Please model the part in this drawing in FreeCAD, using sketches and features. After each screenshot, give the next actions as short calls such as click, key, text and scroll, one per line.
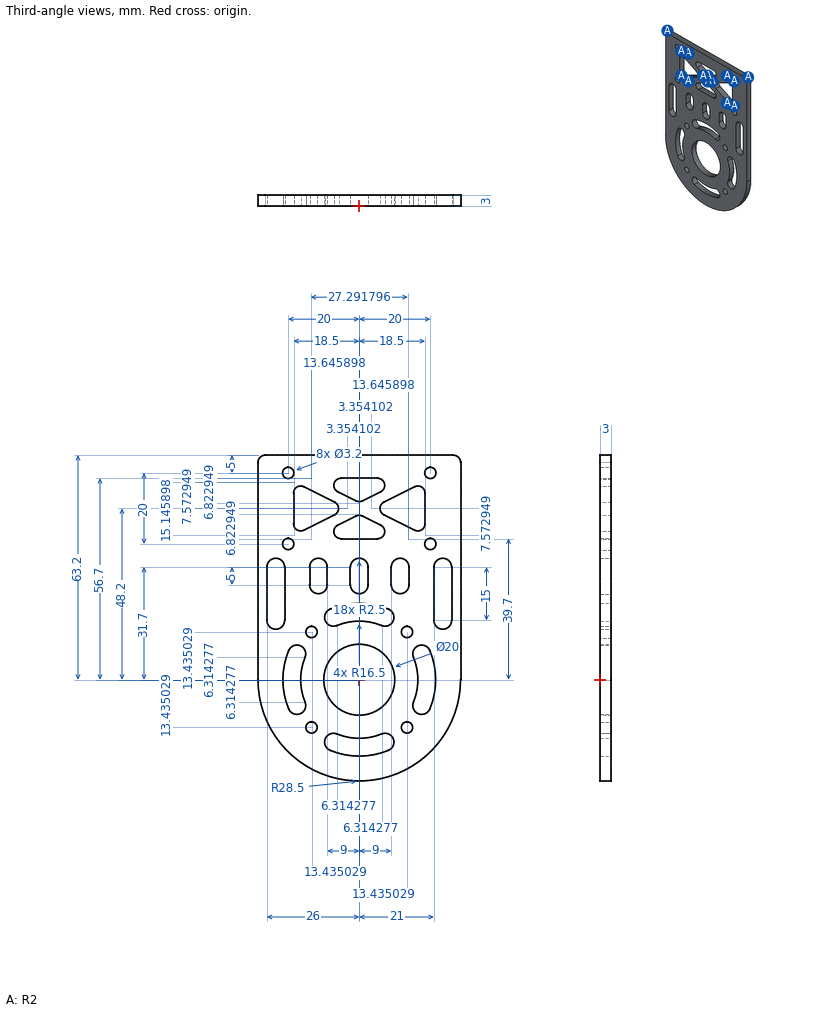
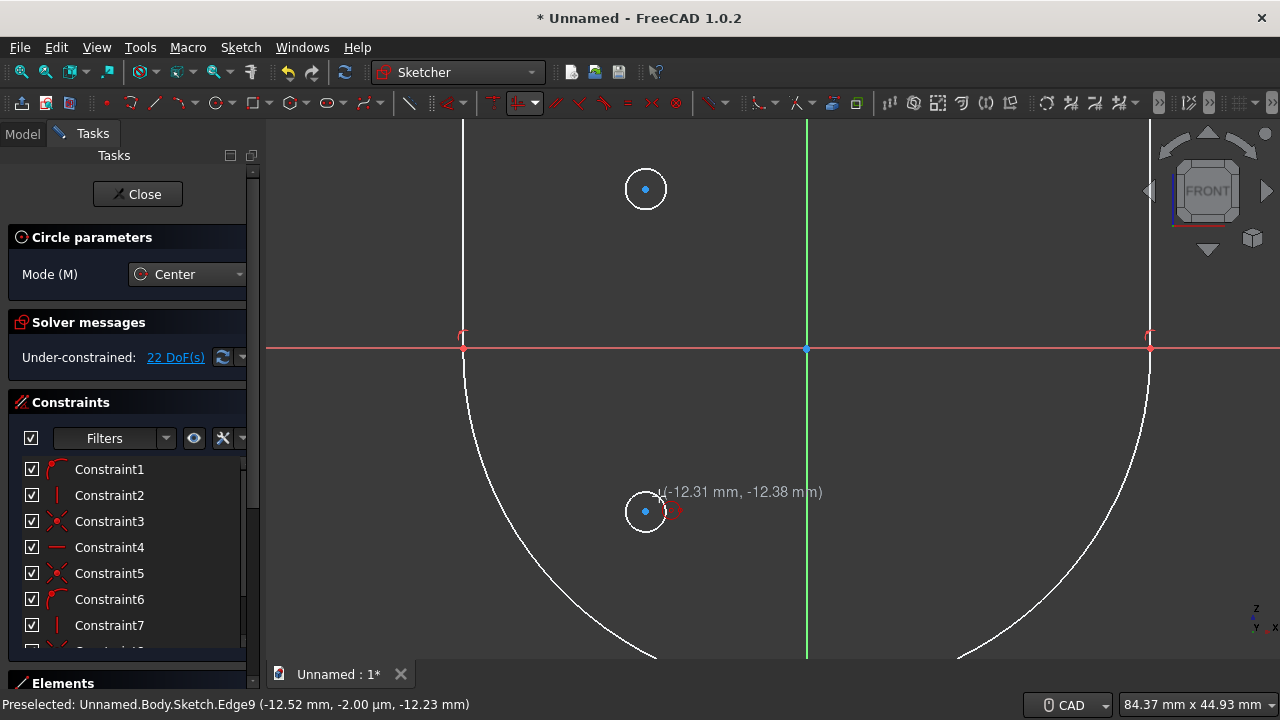
click(968, 187)
click(982, 173)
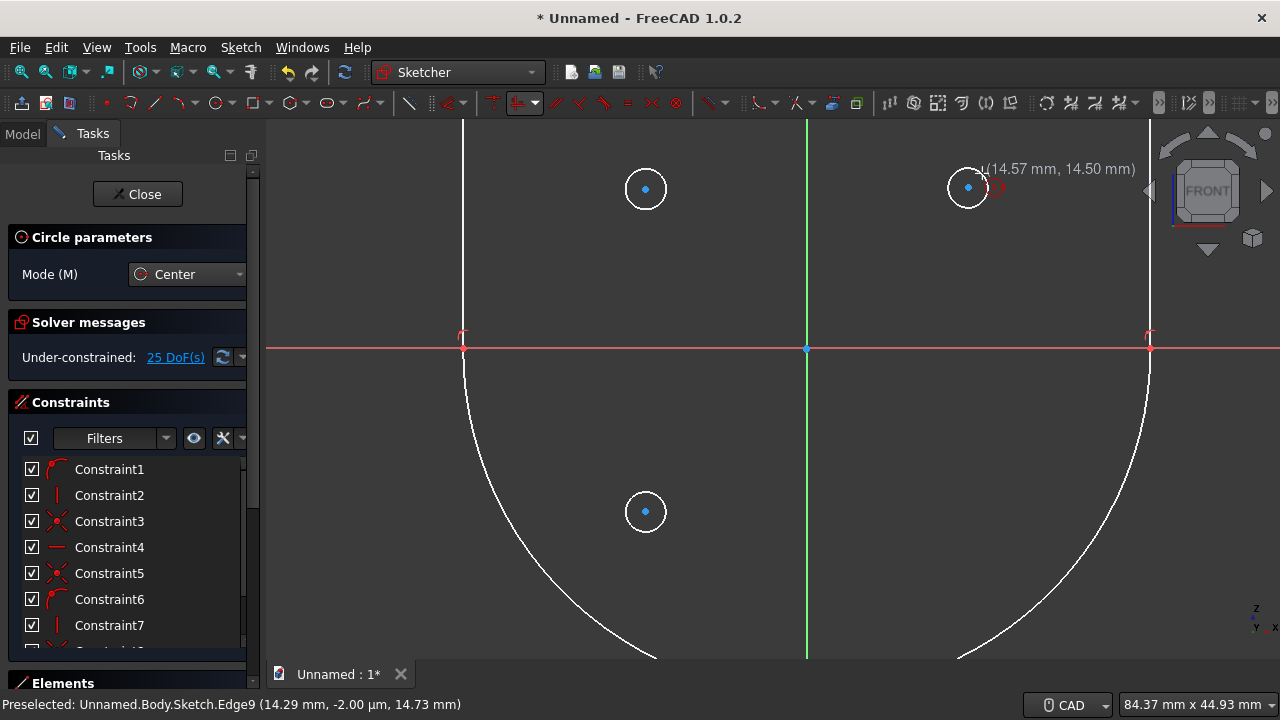
click(807, 348)
click(892, 263)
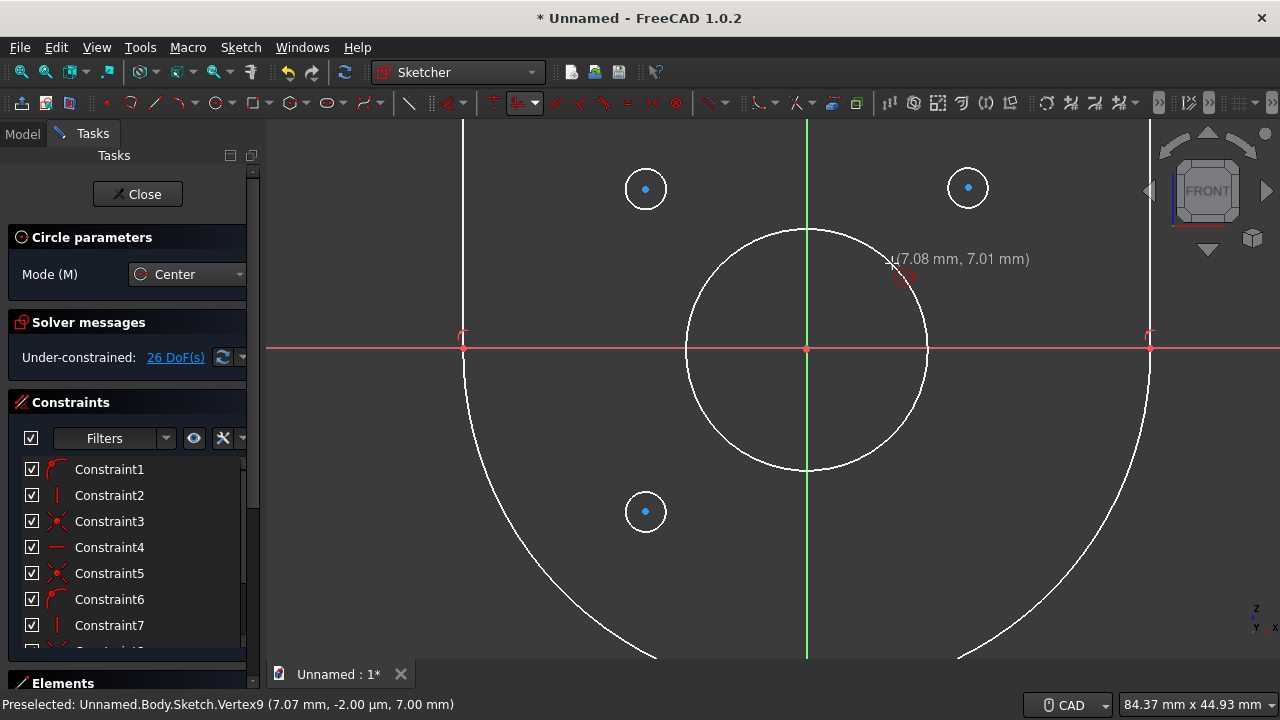
click(968, 510)
click(982, 496)
key(Escape)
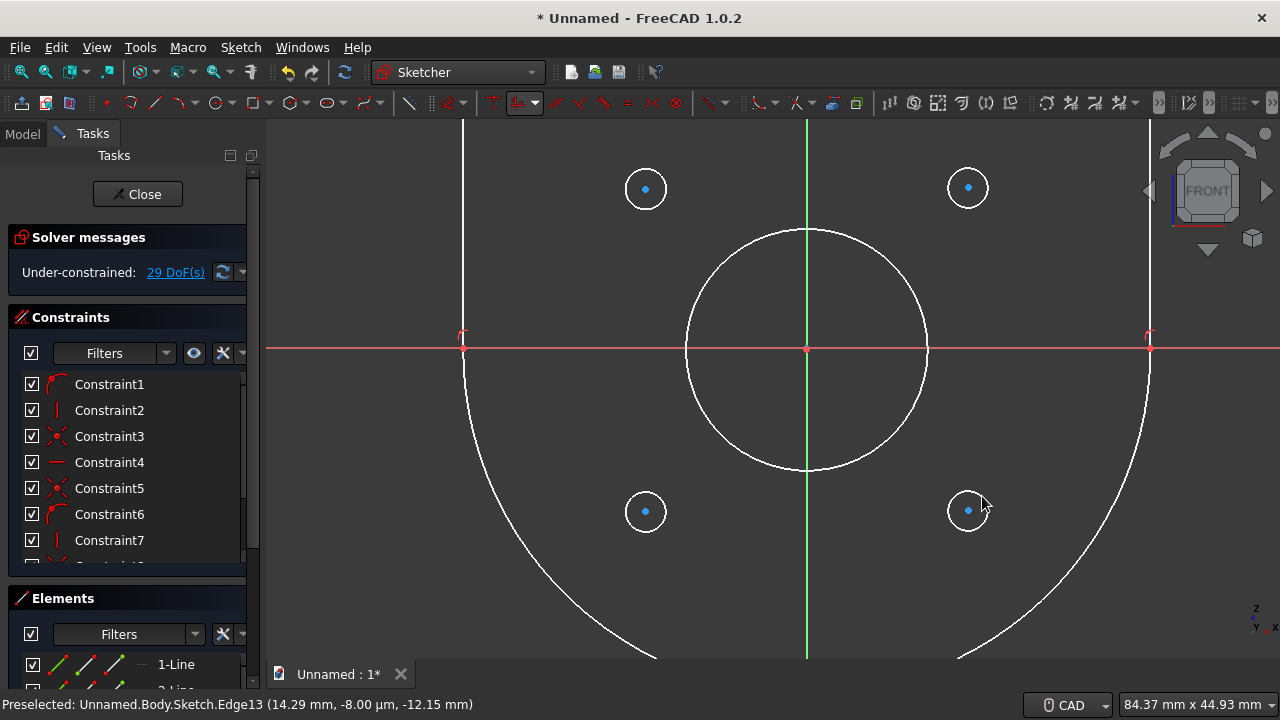
scroll(807, 349, up, 4)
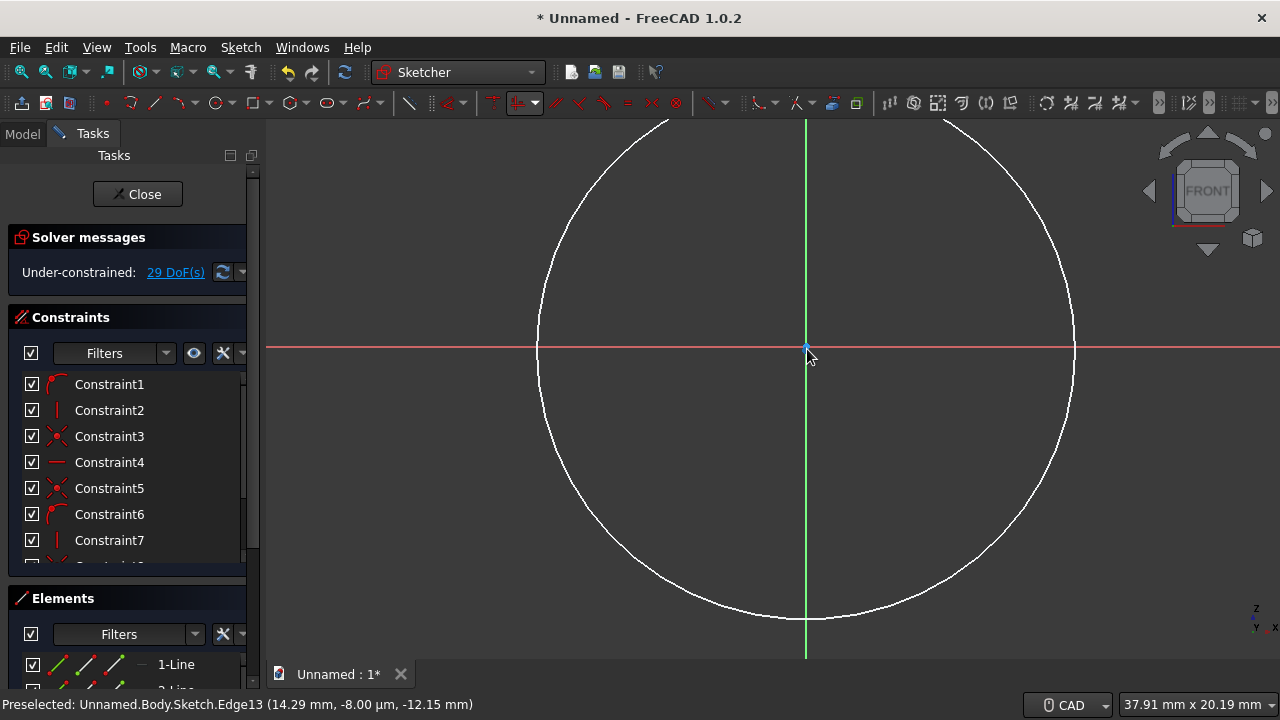
drag(796, 337, 816, 360)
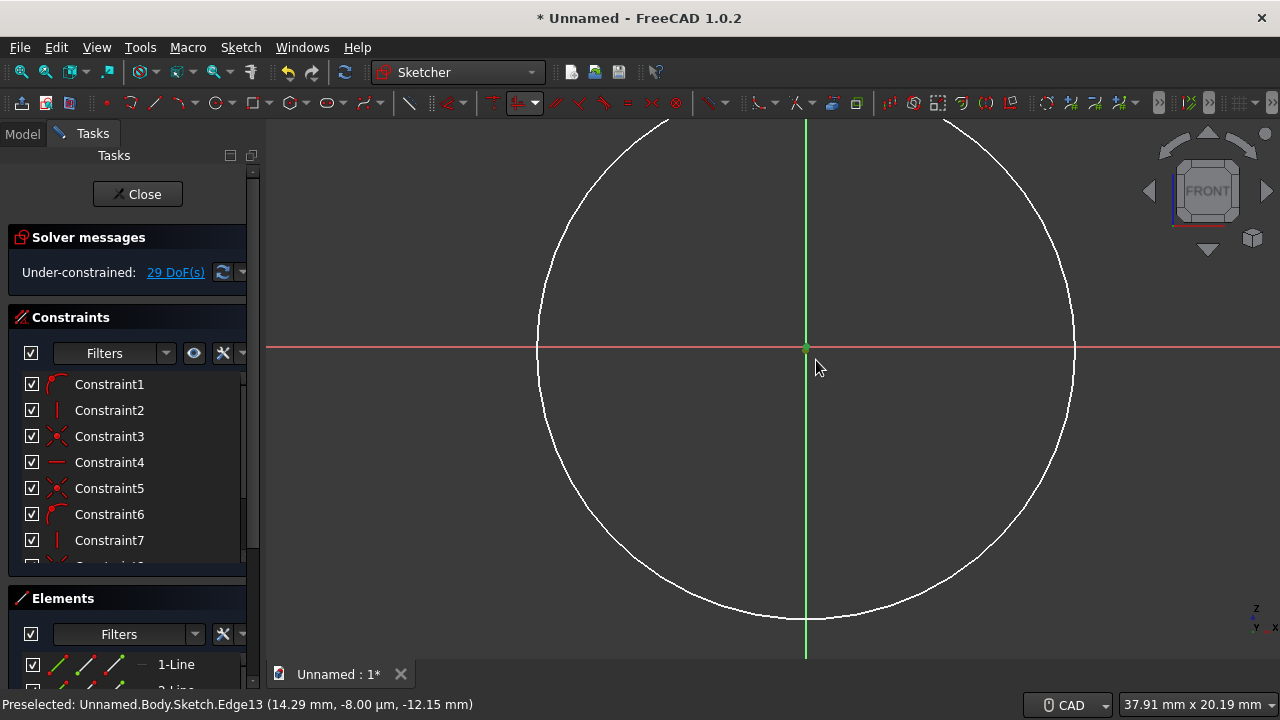
key(c)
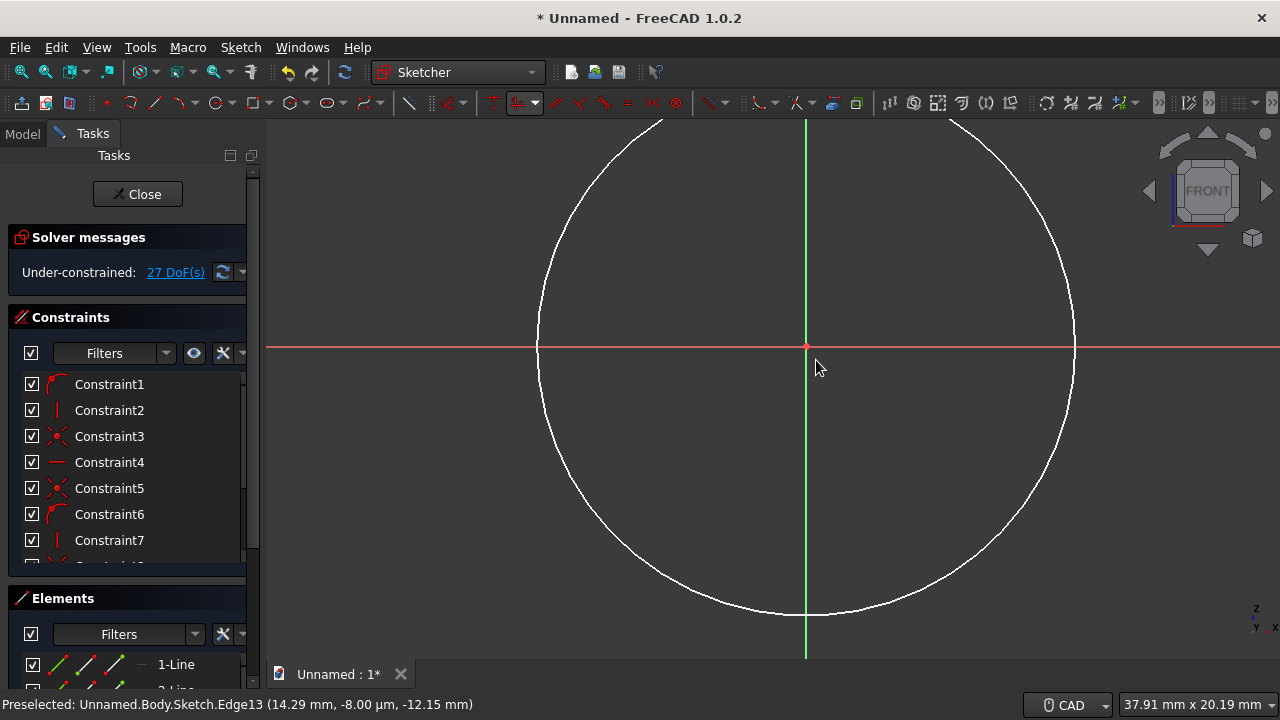
scroll(689, 468, down, 10)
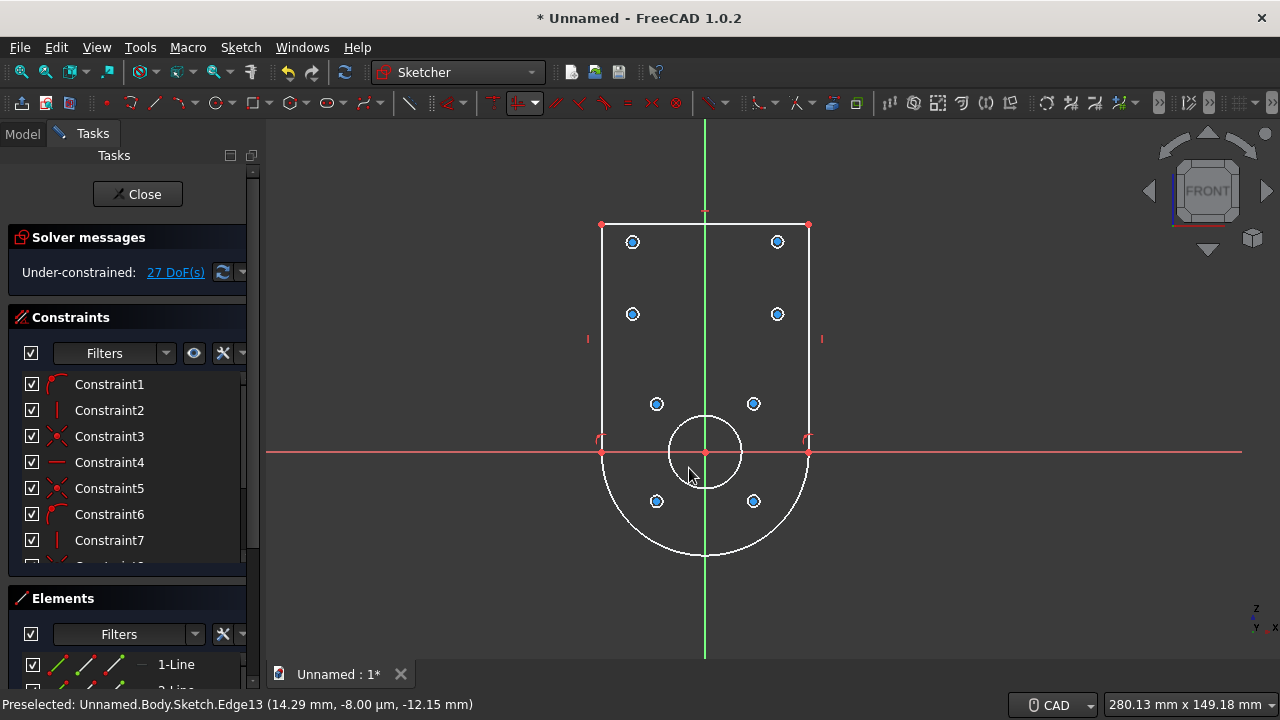
scroll(637, 238, up, 4)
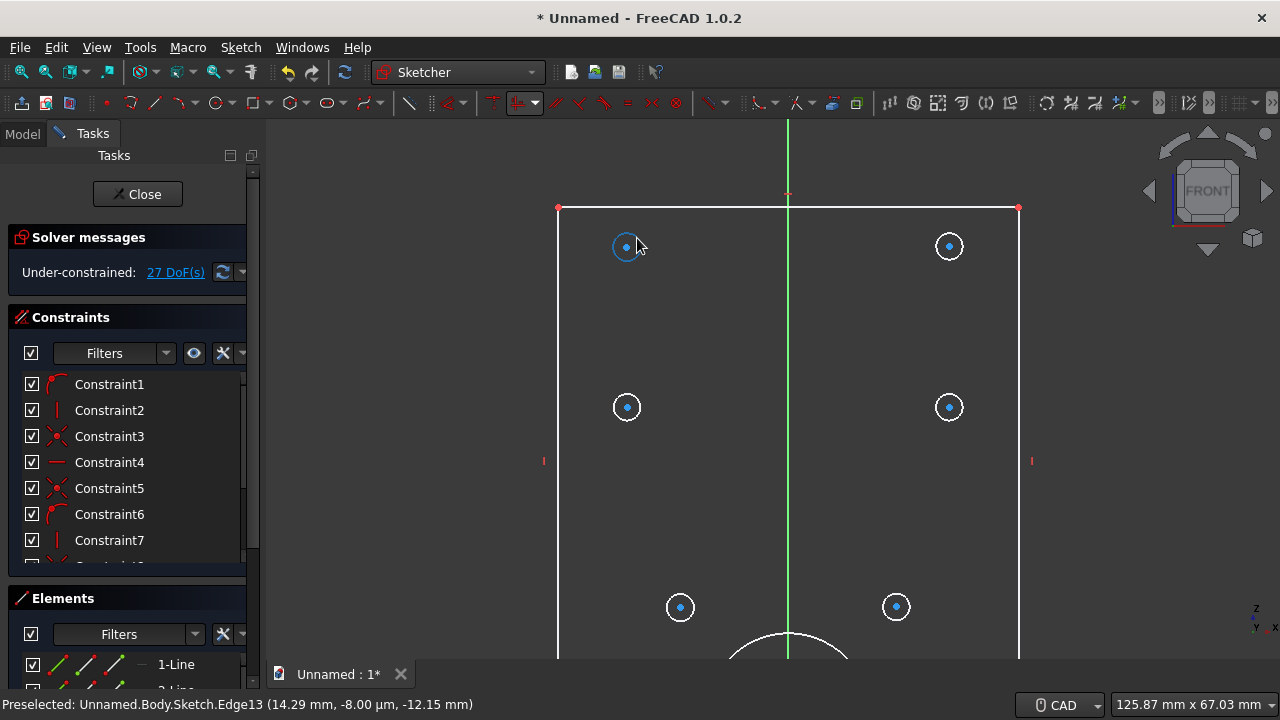
click(637, 237)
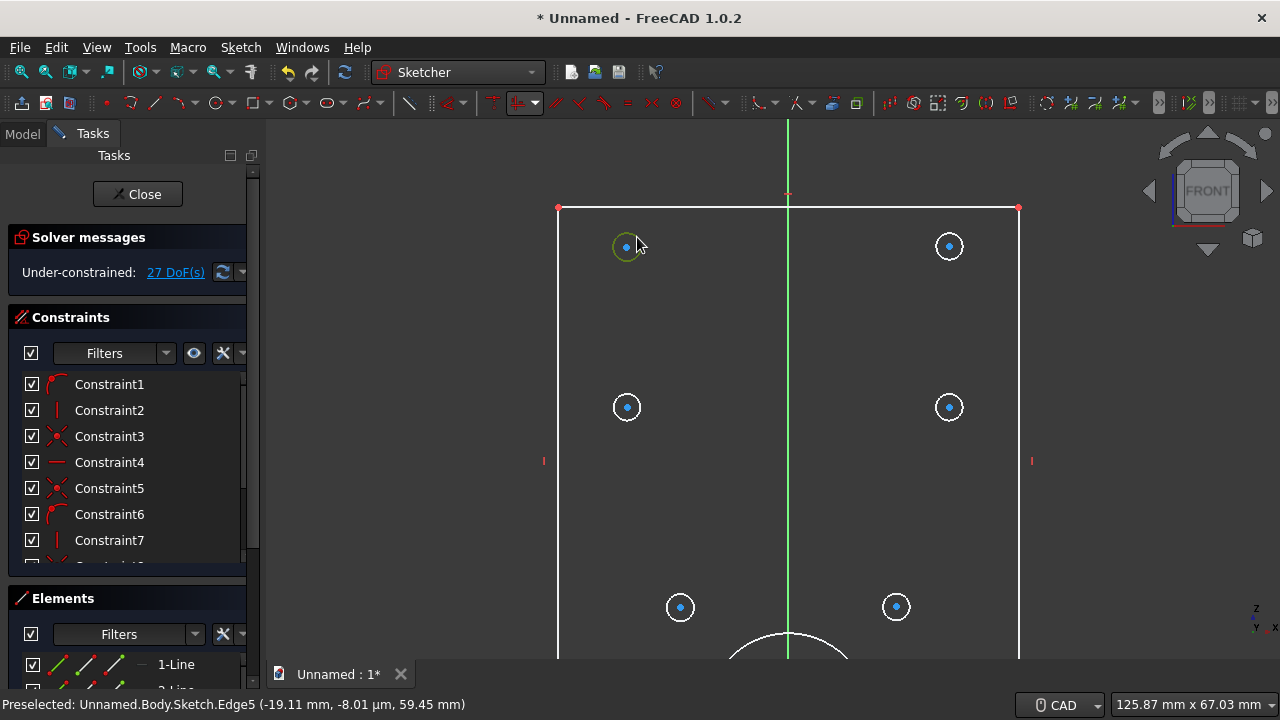
click(636, 398)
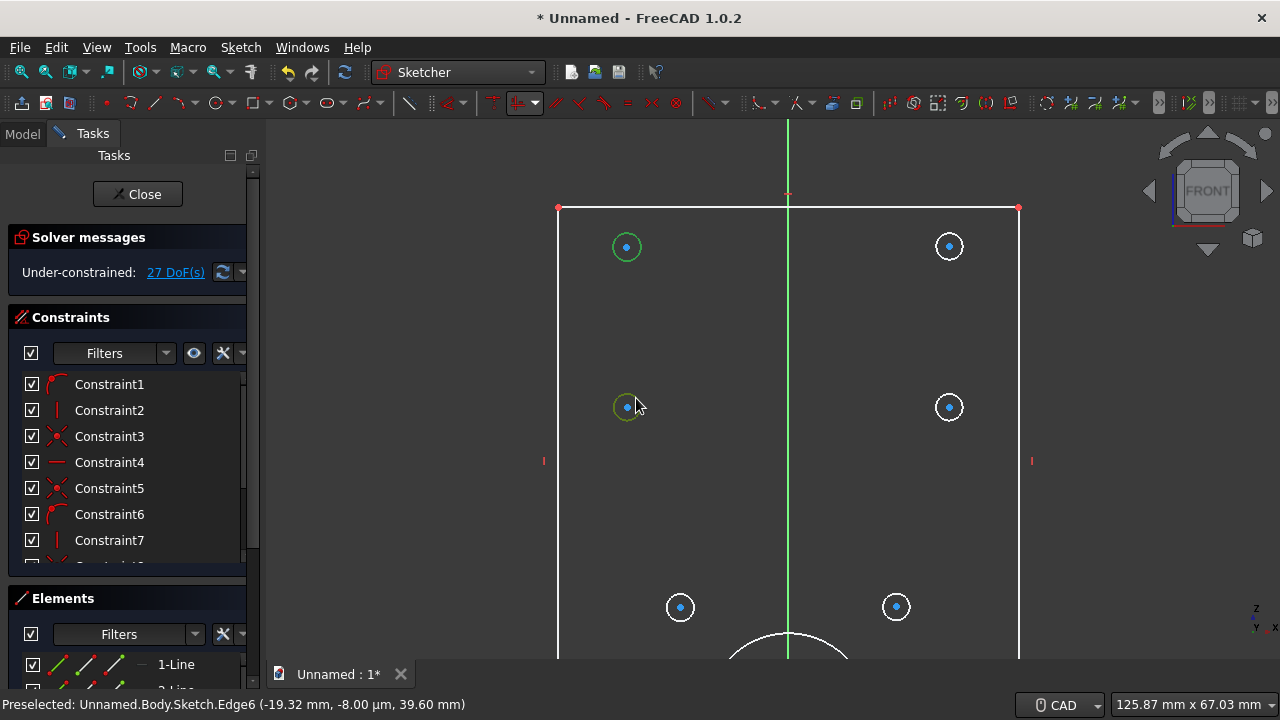
click(959, 237)